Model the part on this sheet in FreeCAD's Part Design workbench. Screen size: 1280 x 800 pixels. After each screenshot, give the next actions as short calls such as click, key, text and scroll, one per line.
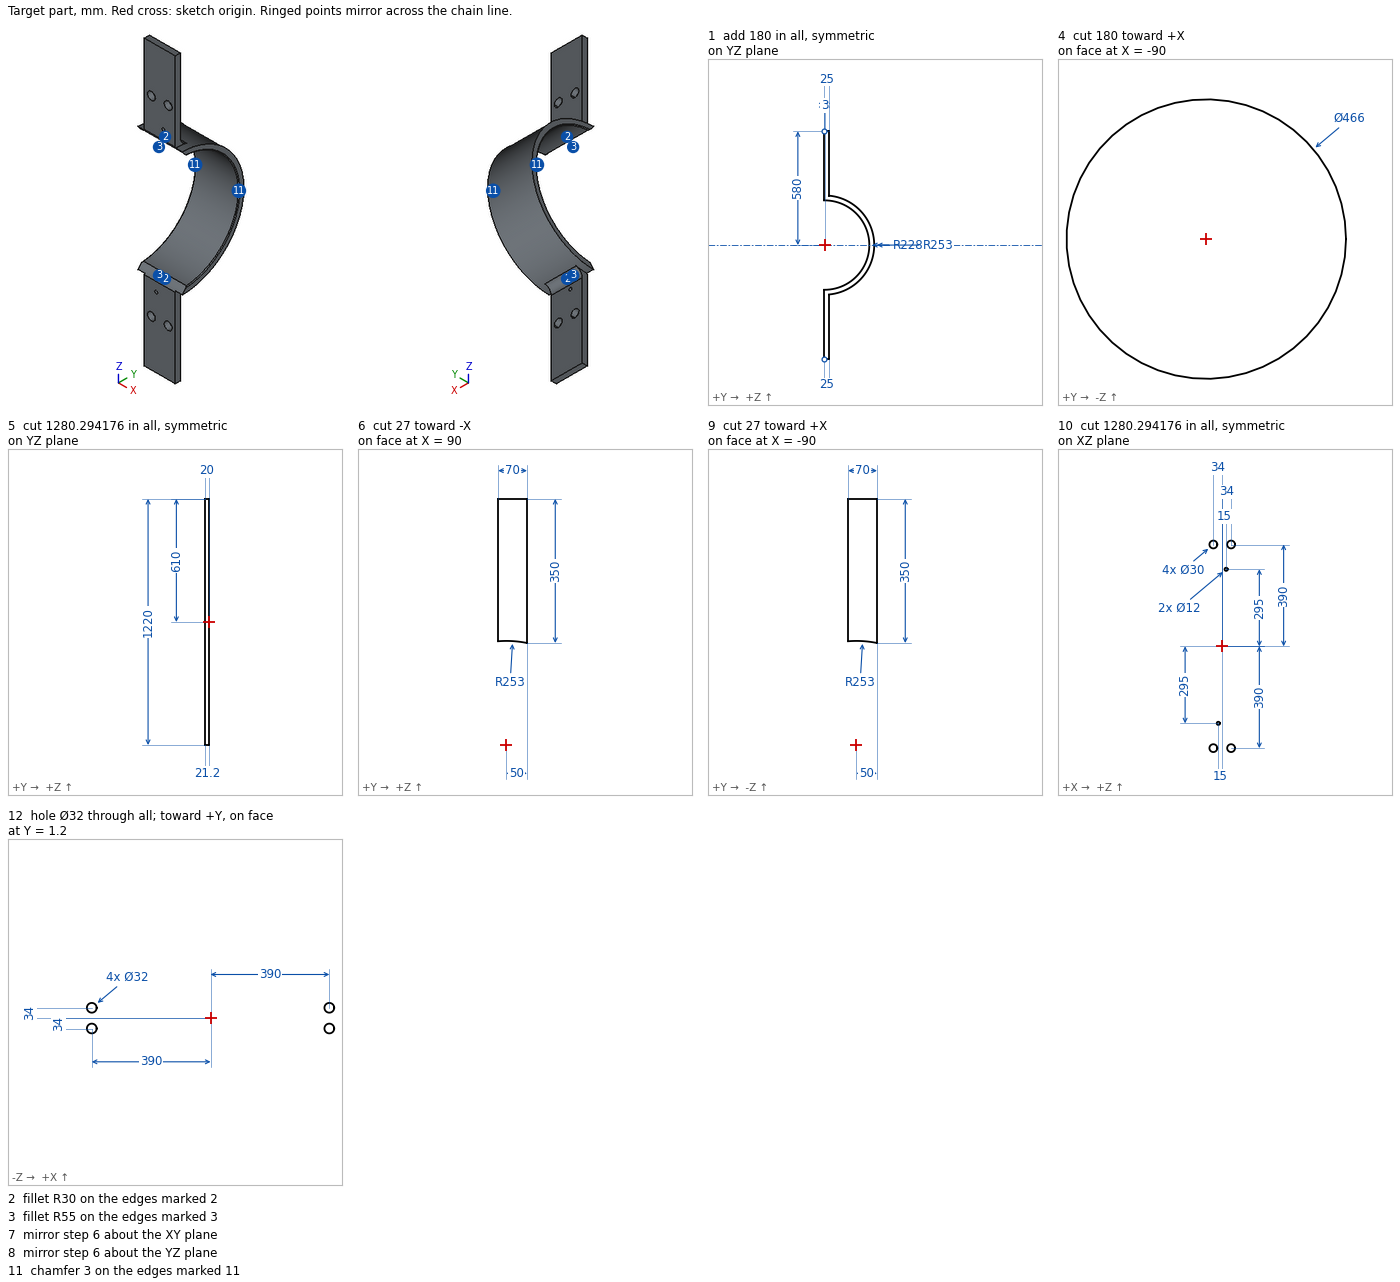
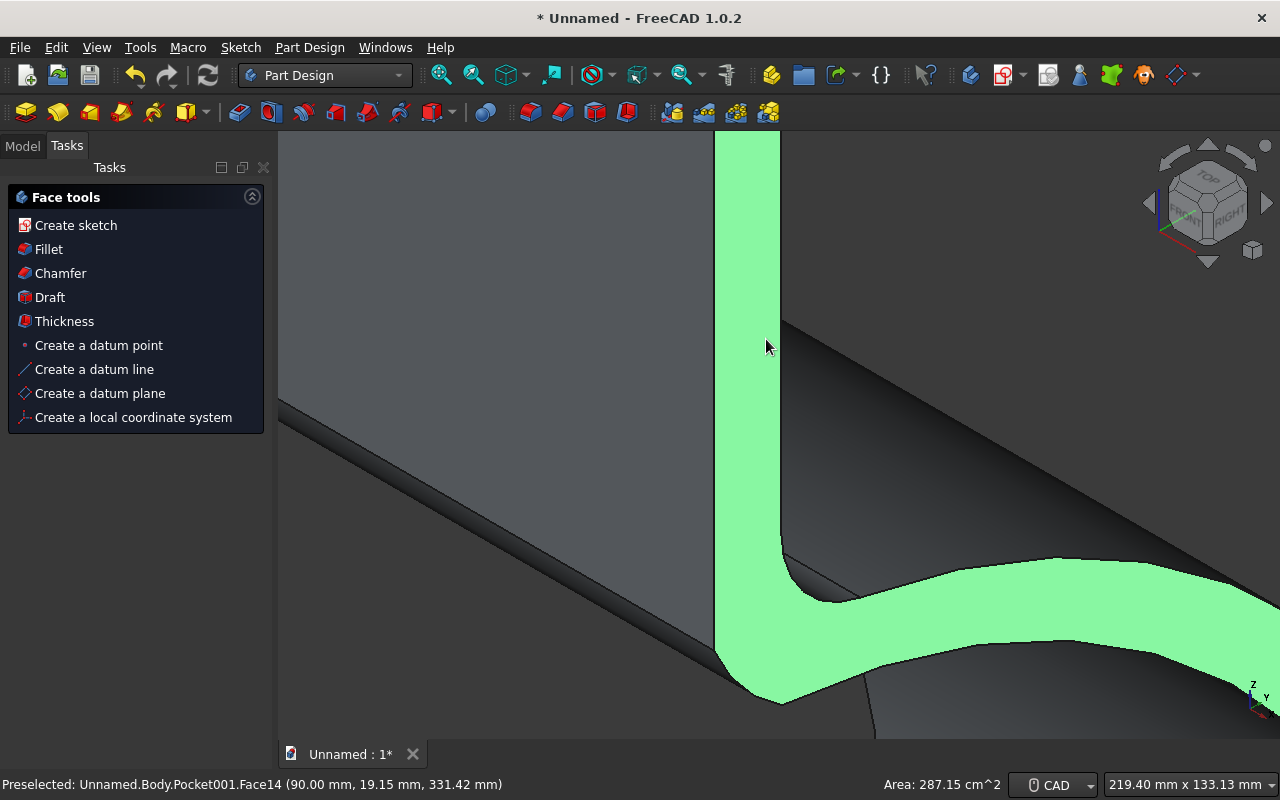
click(1004, 76)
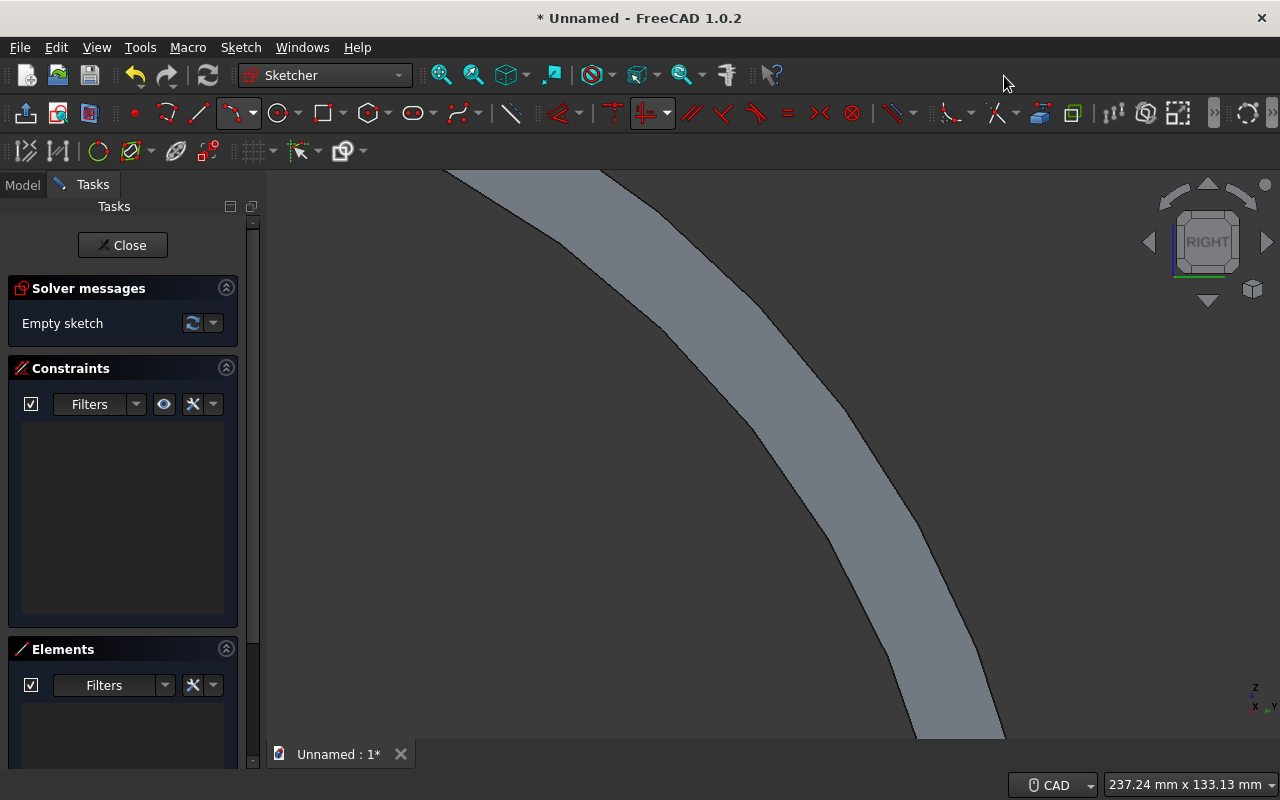
scroll(809, 562, down, 10)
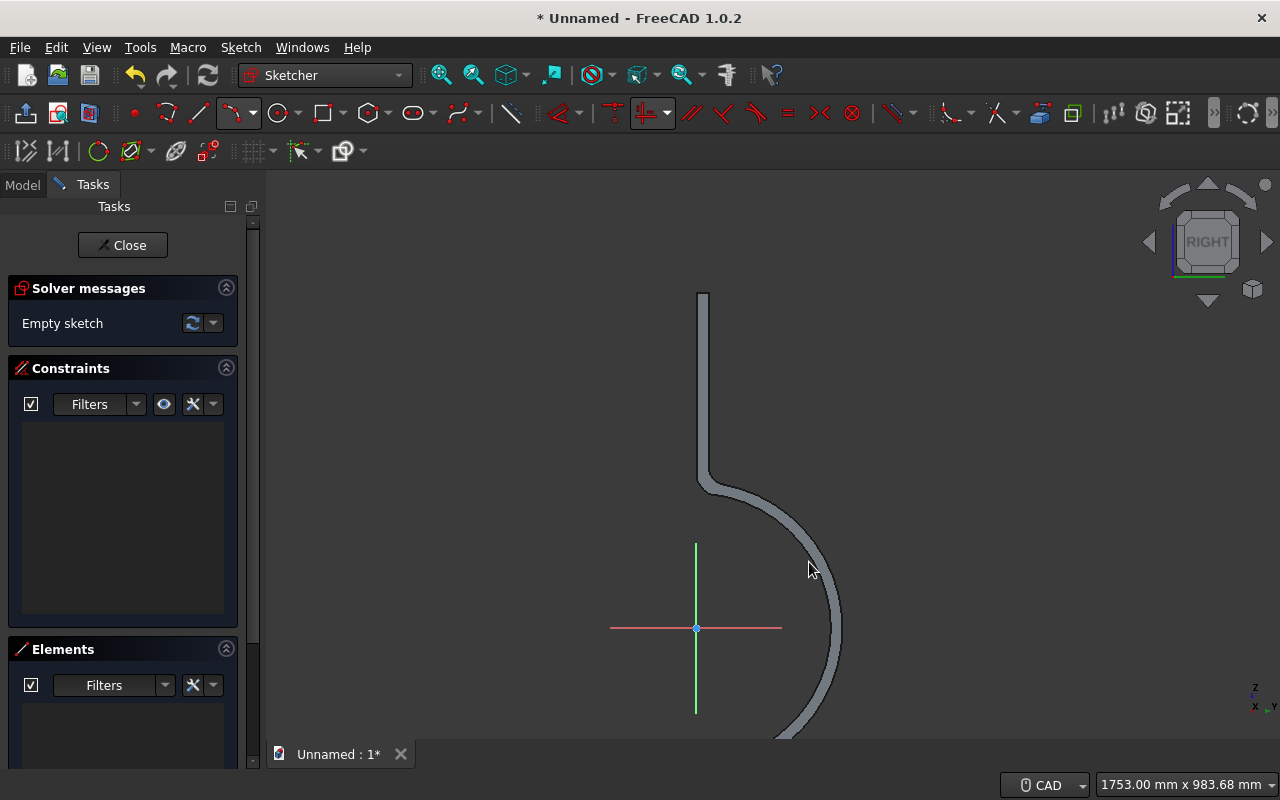
click(168, 114)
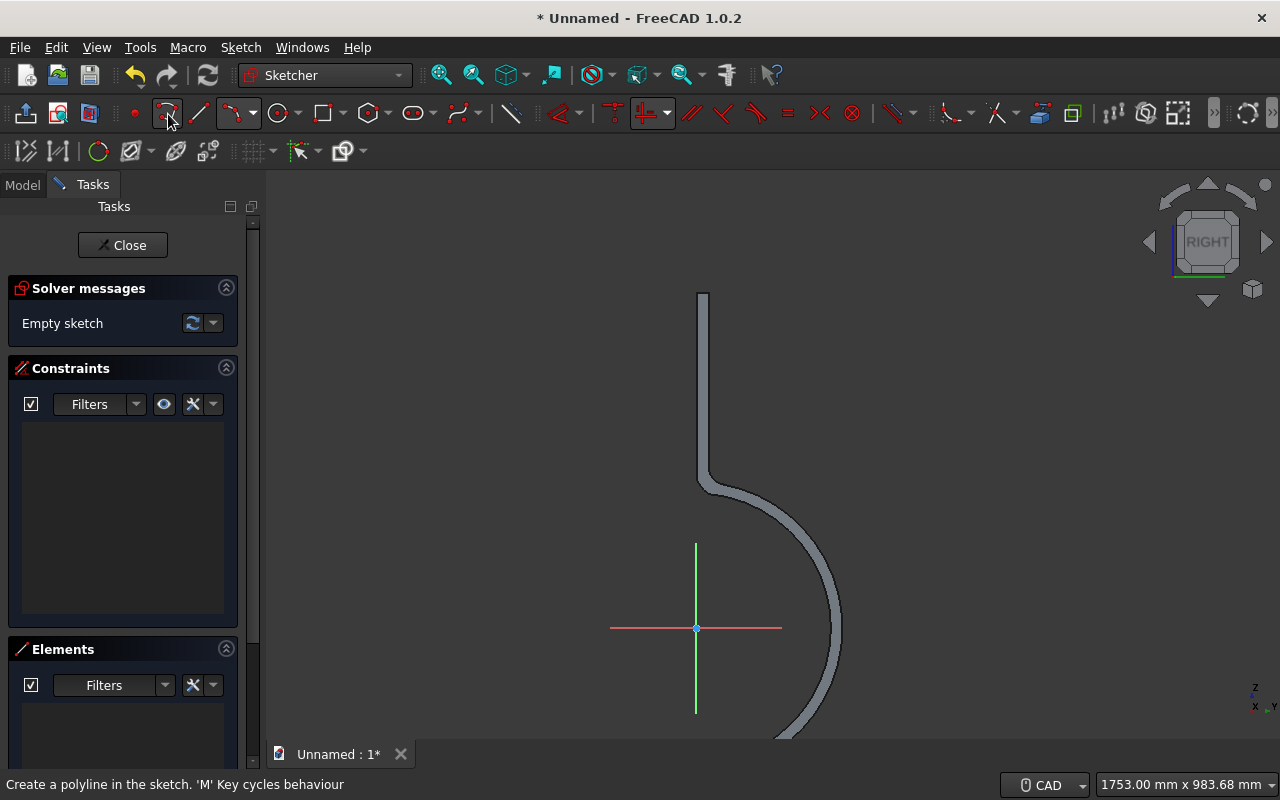
click(725, 485)
click(725, 282)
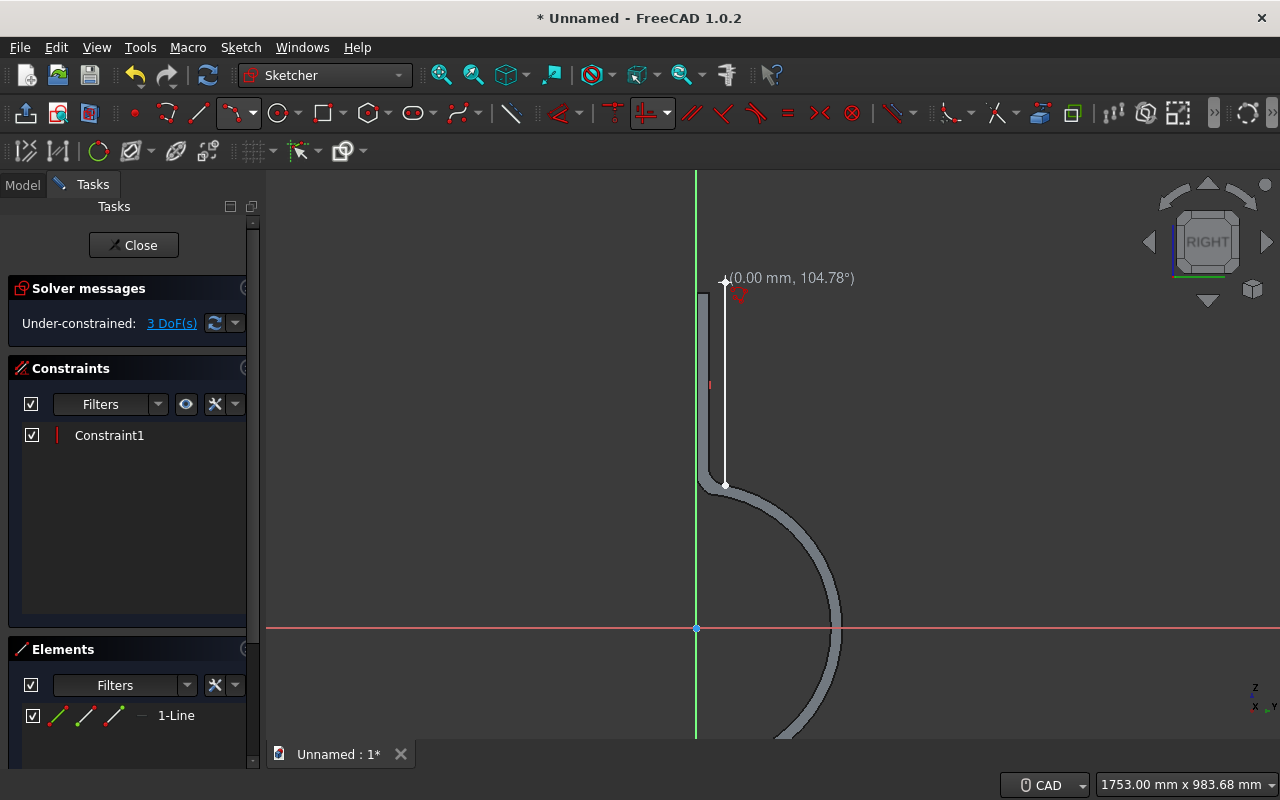
scroll(685, 282, up, 2)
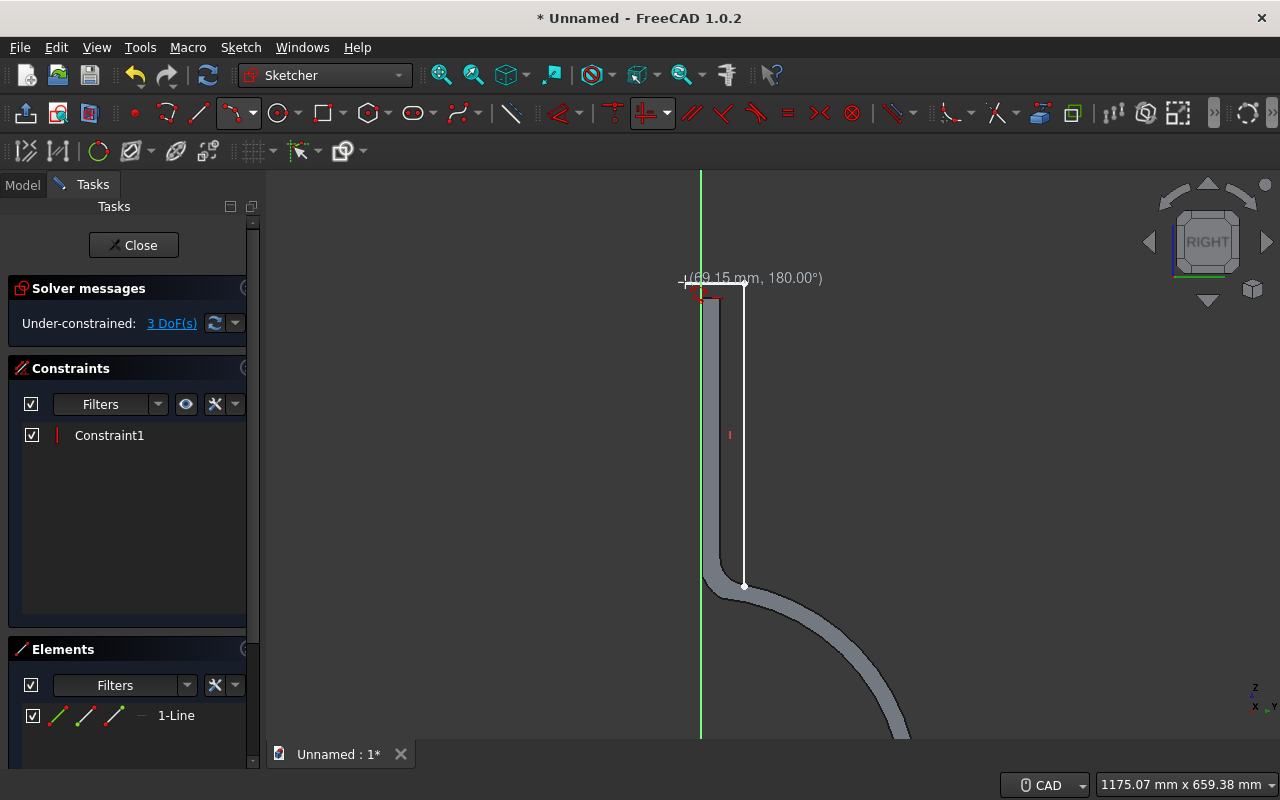
click(684, 282)
click(684, 581)
right_click(684, 581)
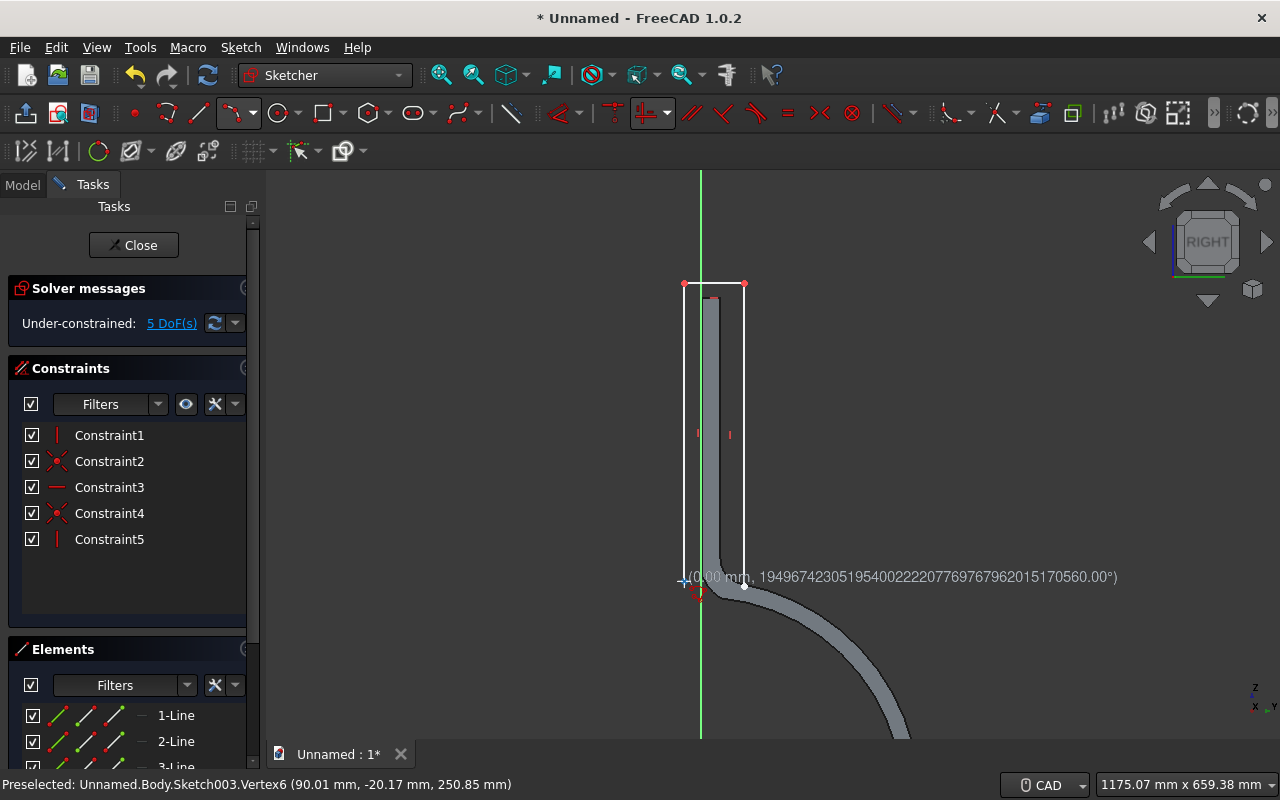
click(232, 114)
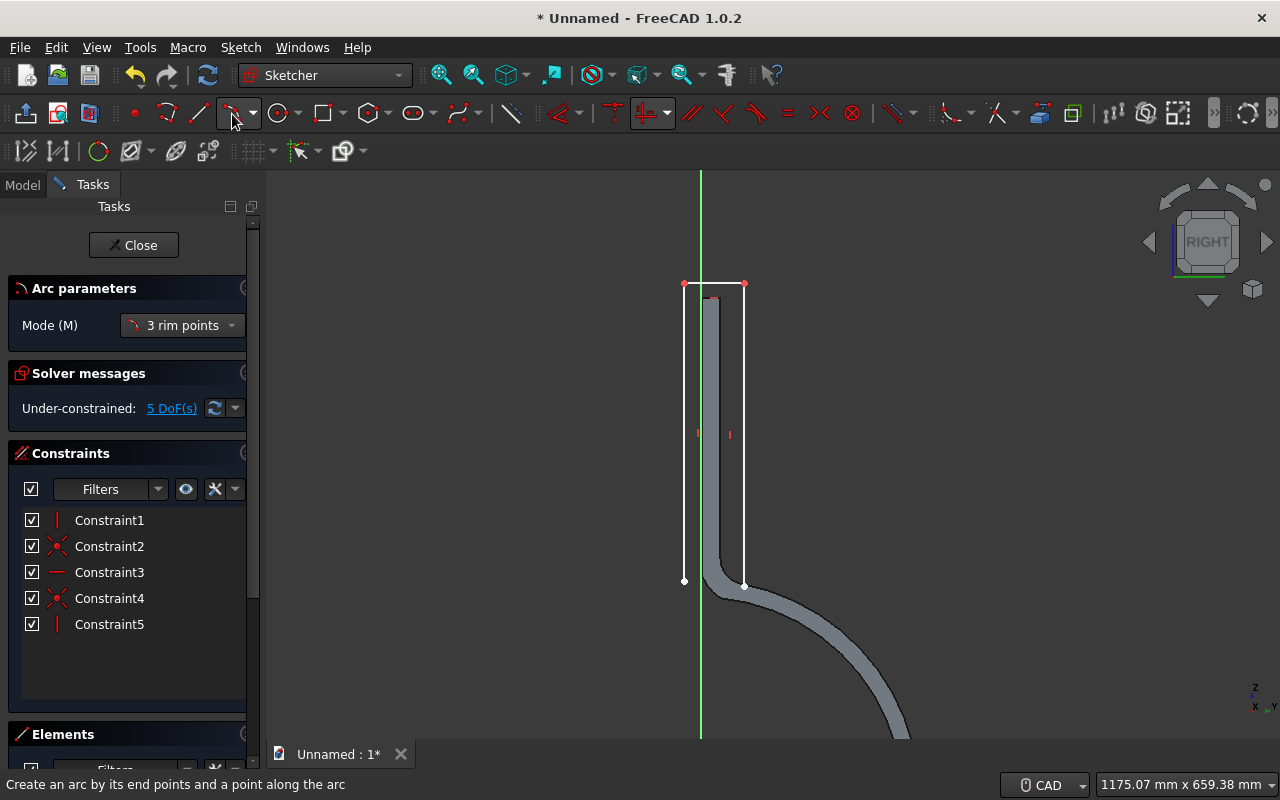
click(684, 582)
click(744, 586)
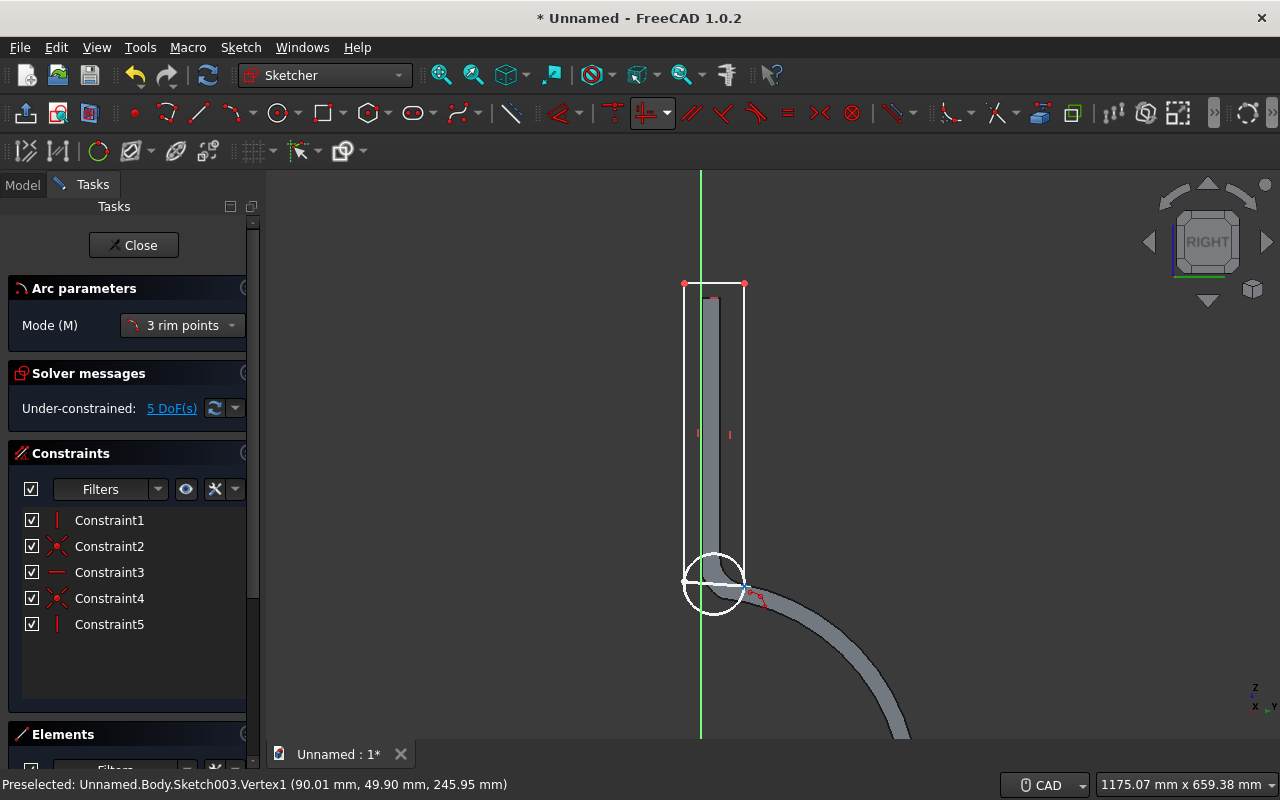
scroll(714, 581, up, 11)